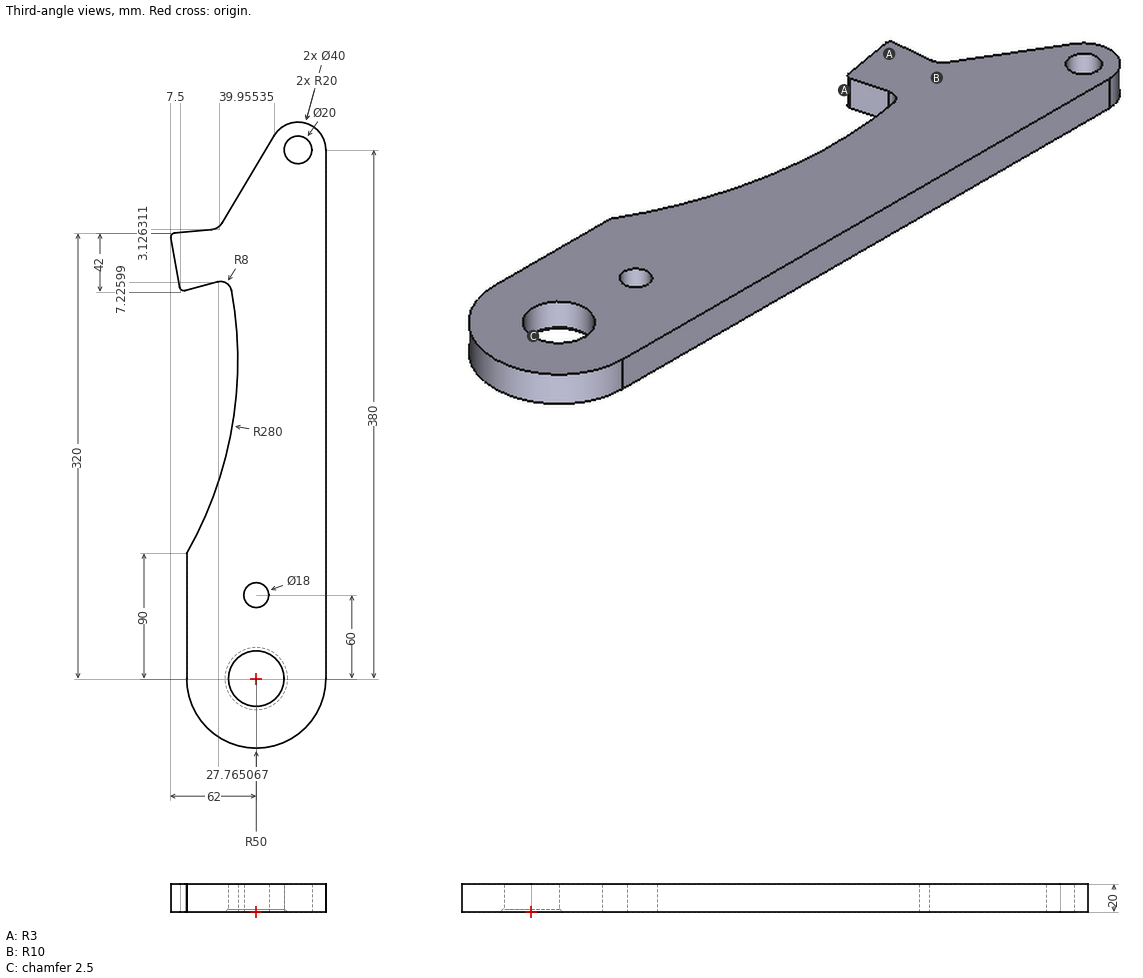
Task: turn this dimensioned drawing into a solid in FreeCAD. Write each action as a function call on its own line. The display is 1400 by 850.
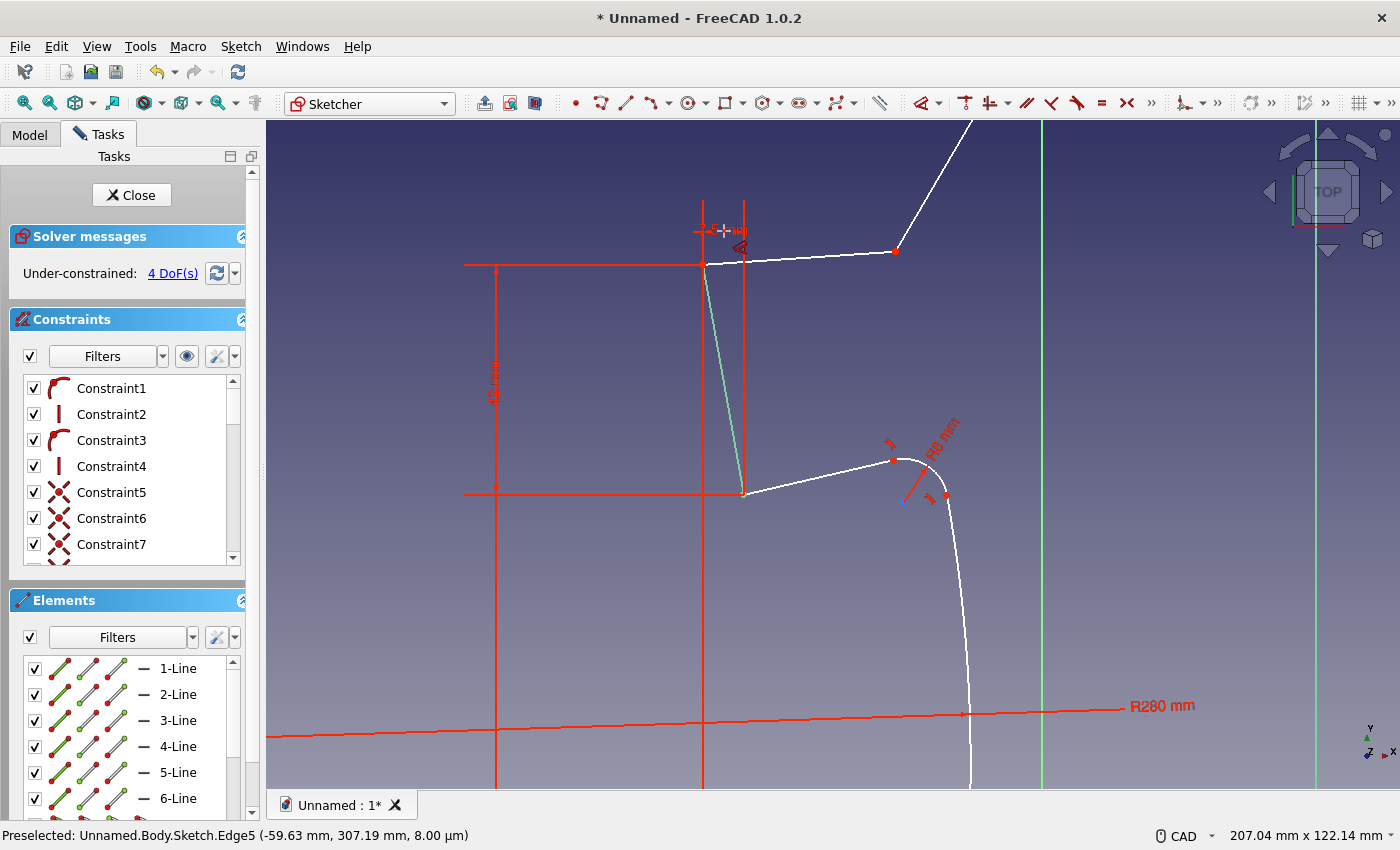
click(789, 484)
click(710, 477)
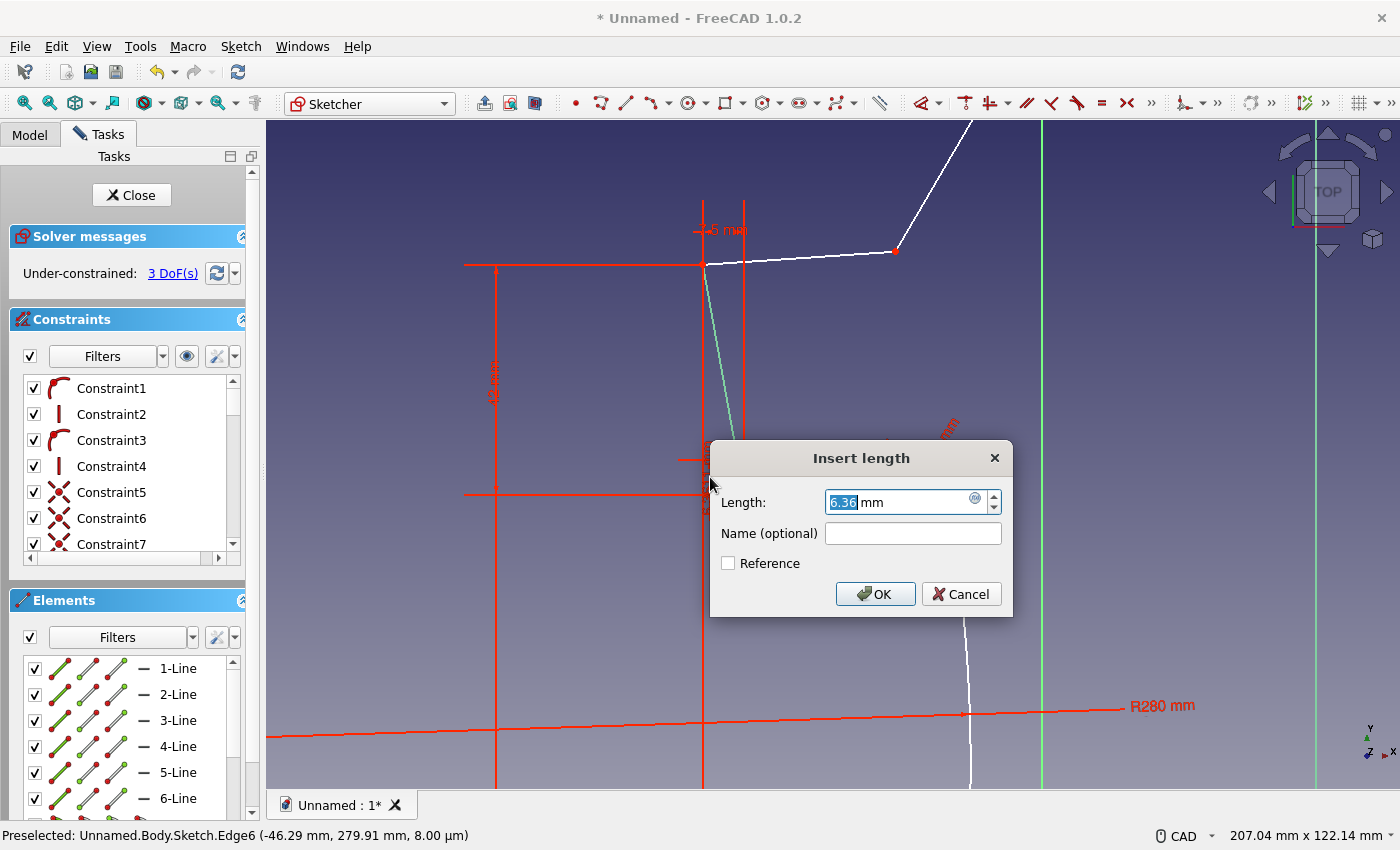
text(7.22599)
key(Return)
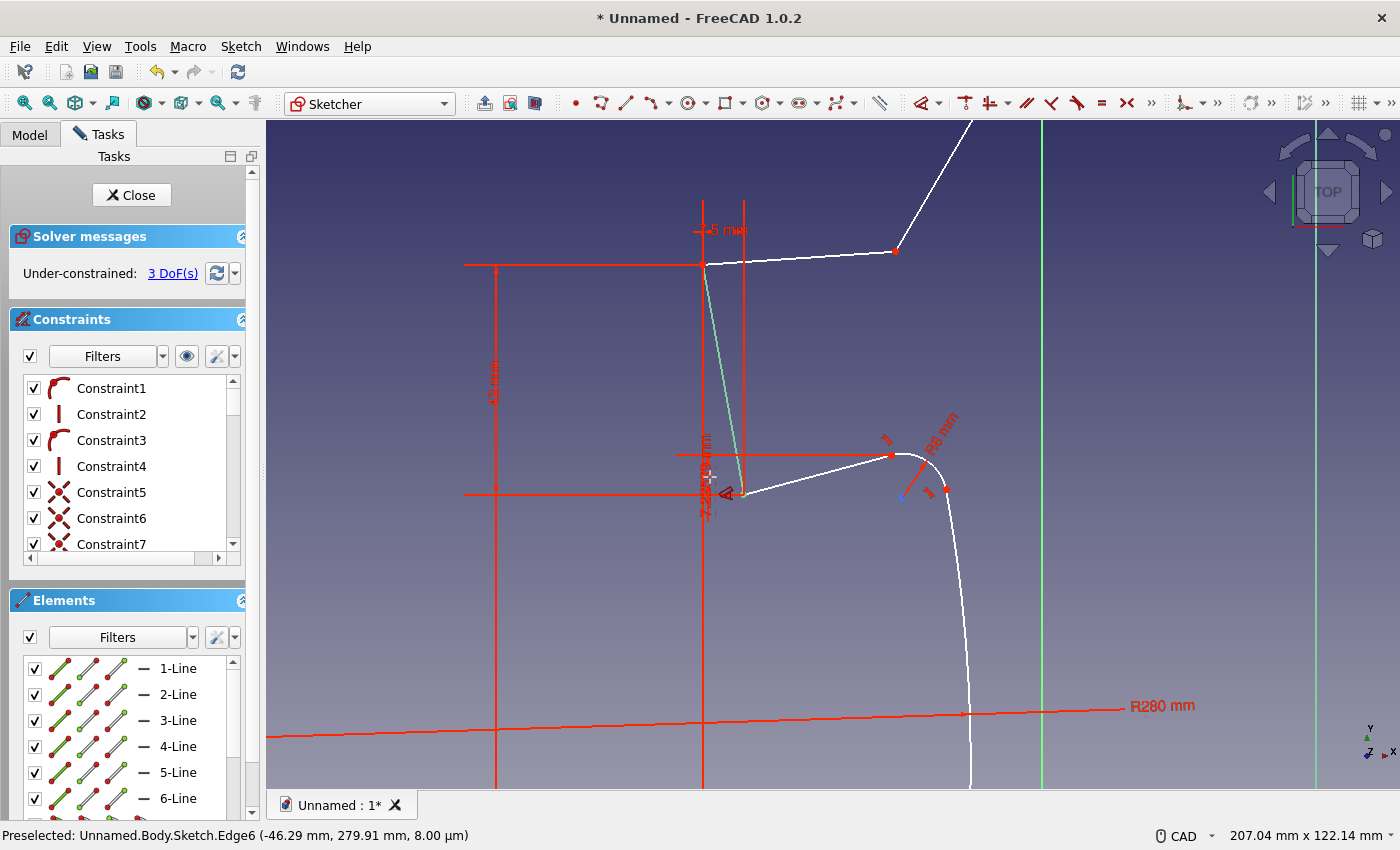
scroll(716, 334, down, 9)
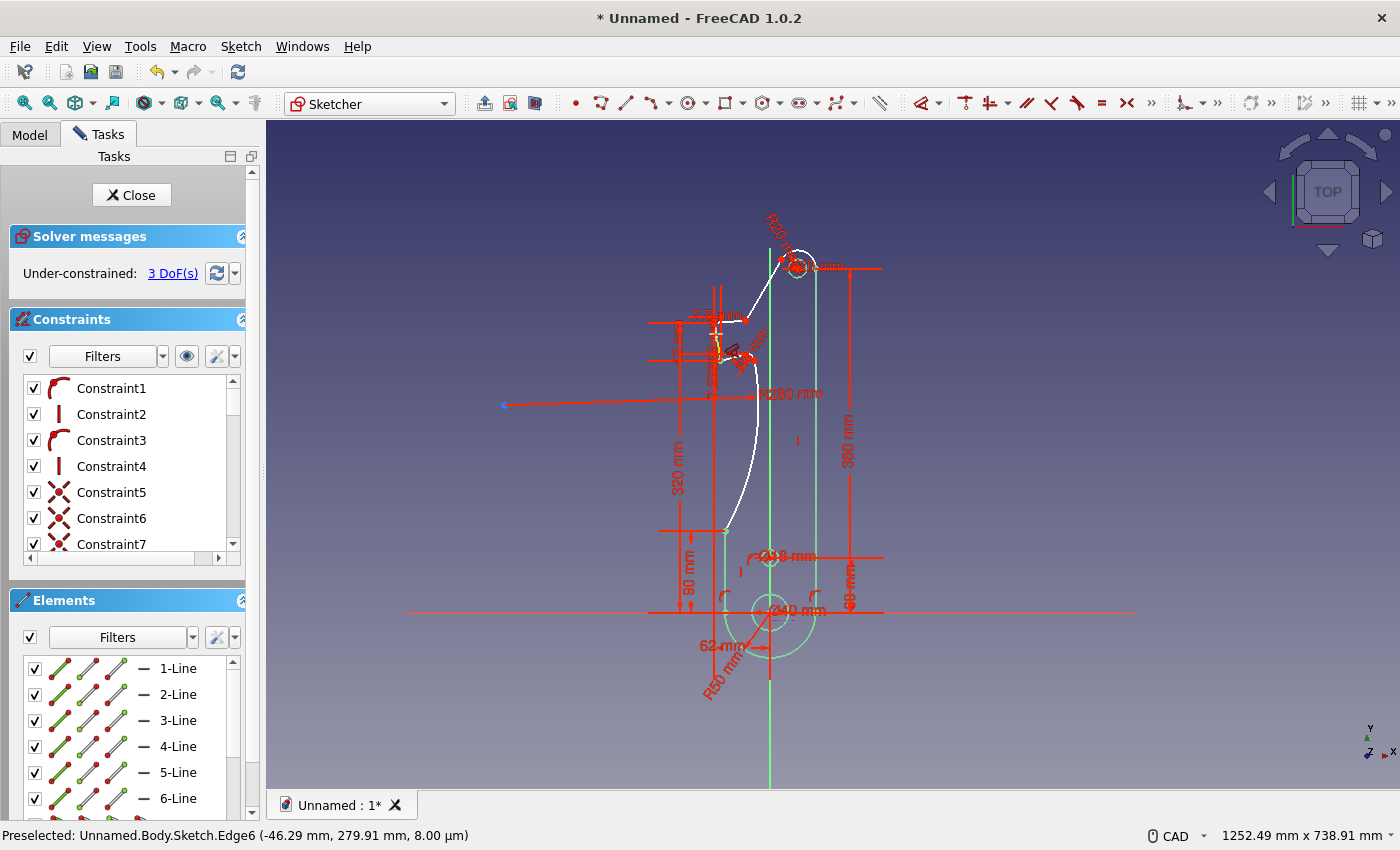
click(753, 308)
click(756, 201)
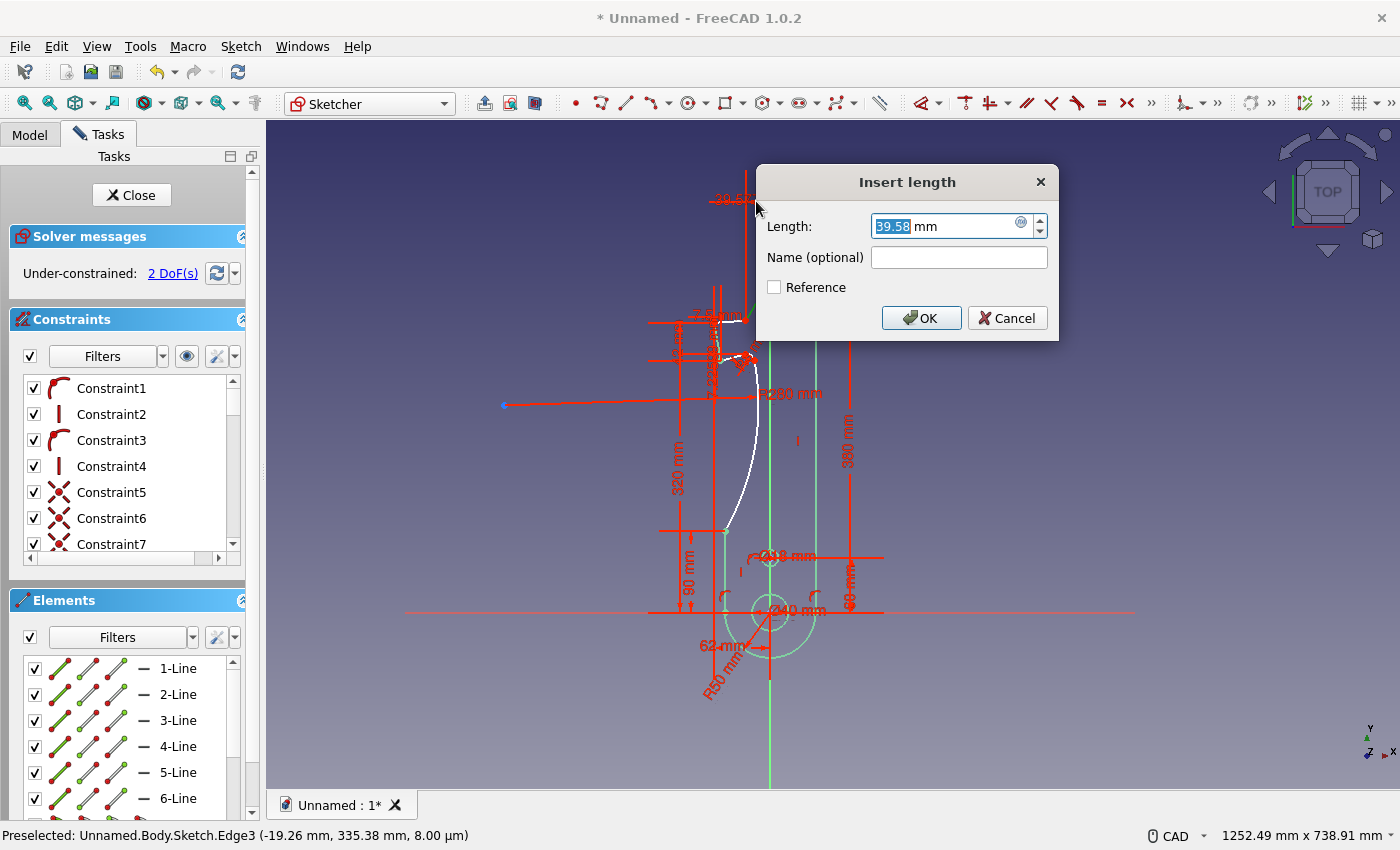
text(39.95535)
key(Return)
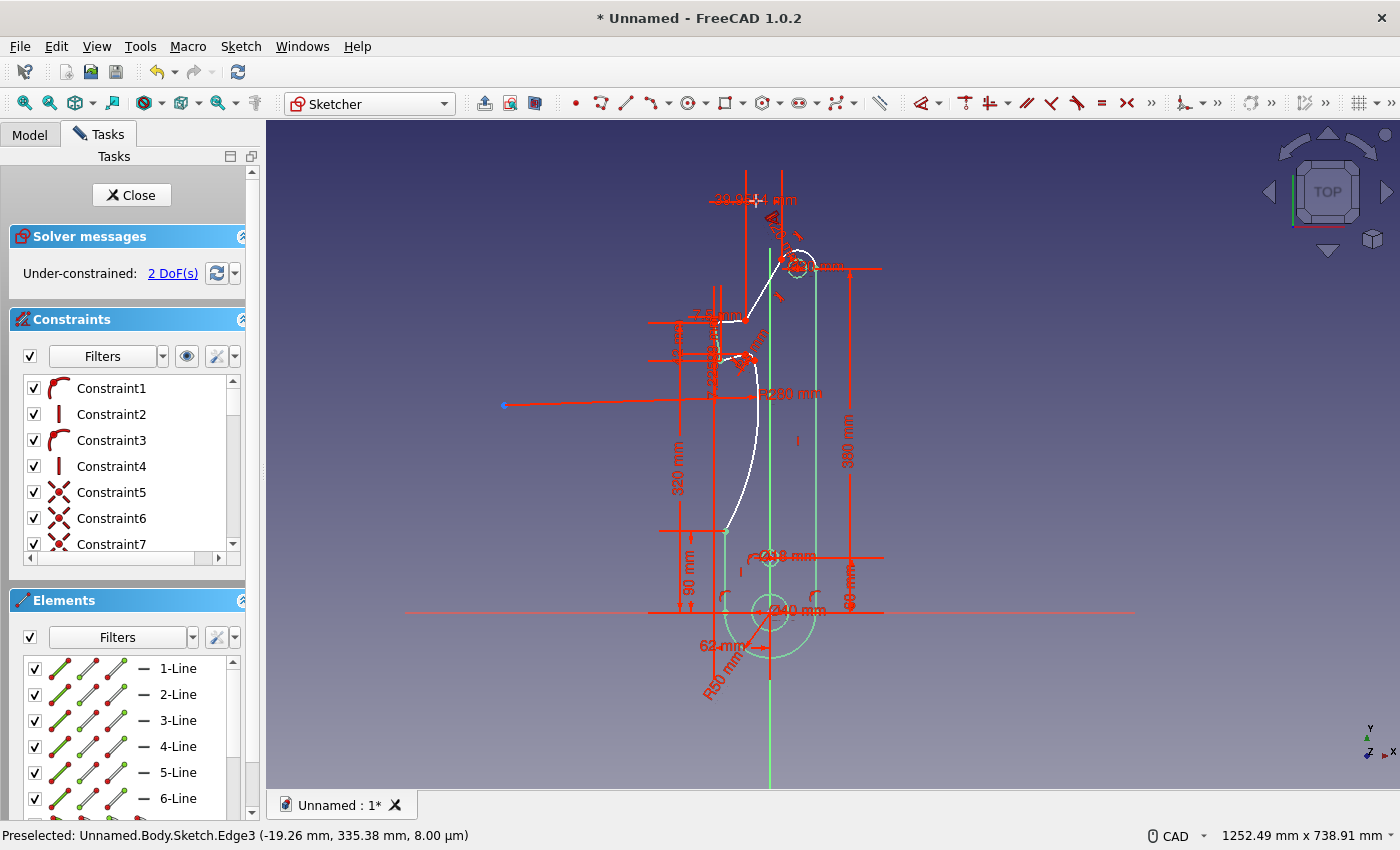
scroll(736, 321, up, 14)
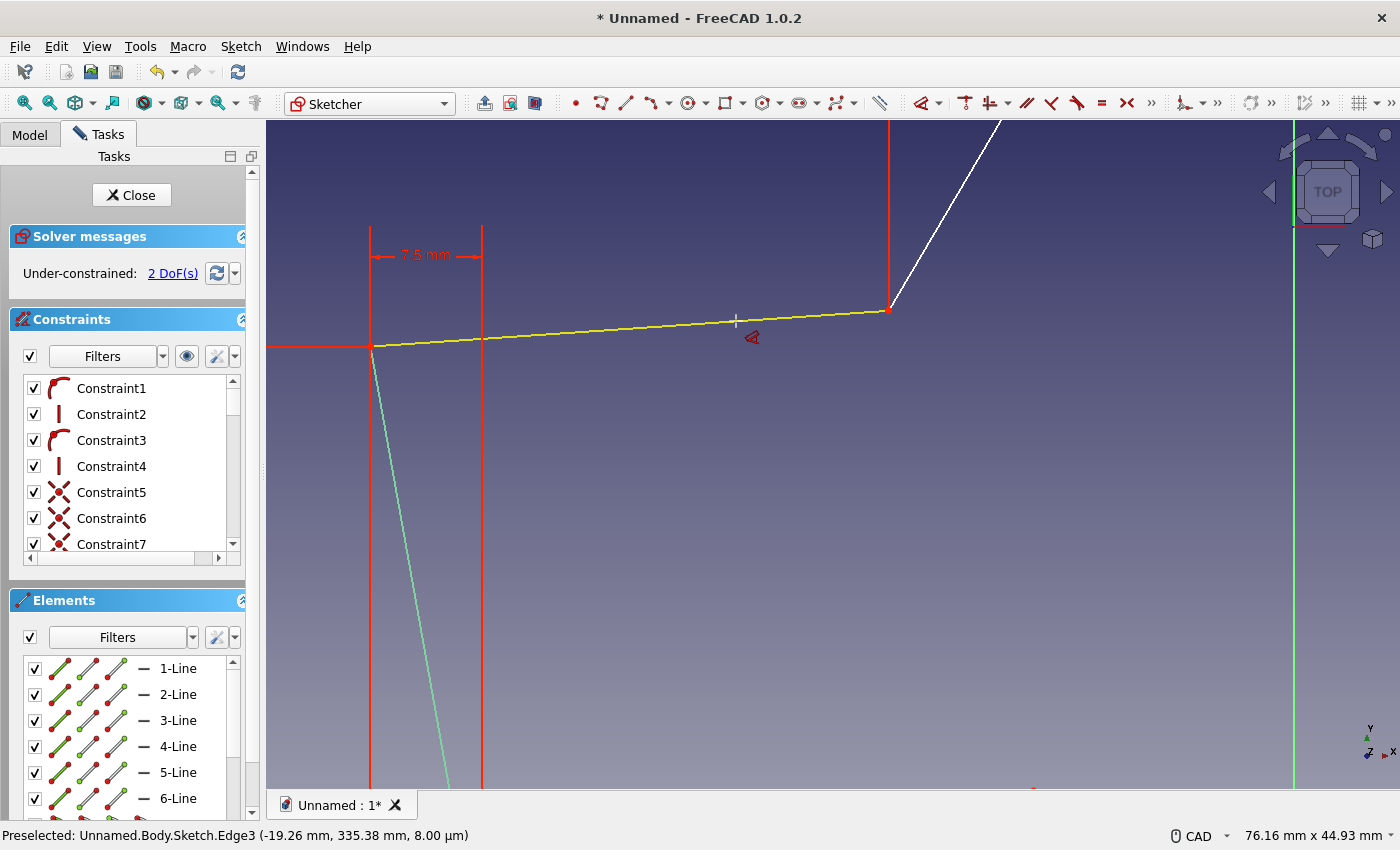
click(733, 322)
click(336, 329)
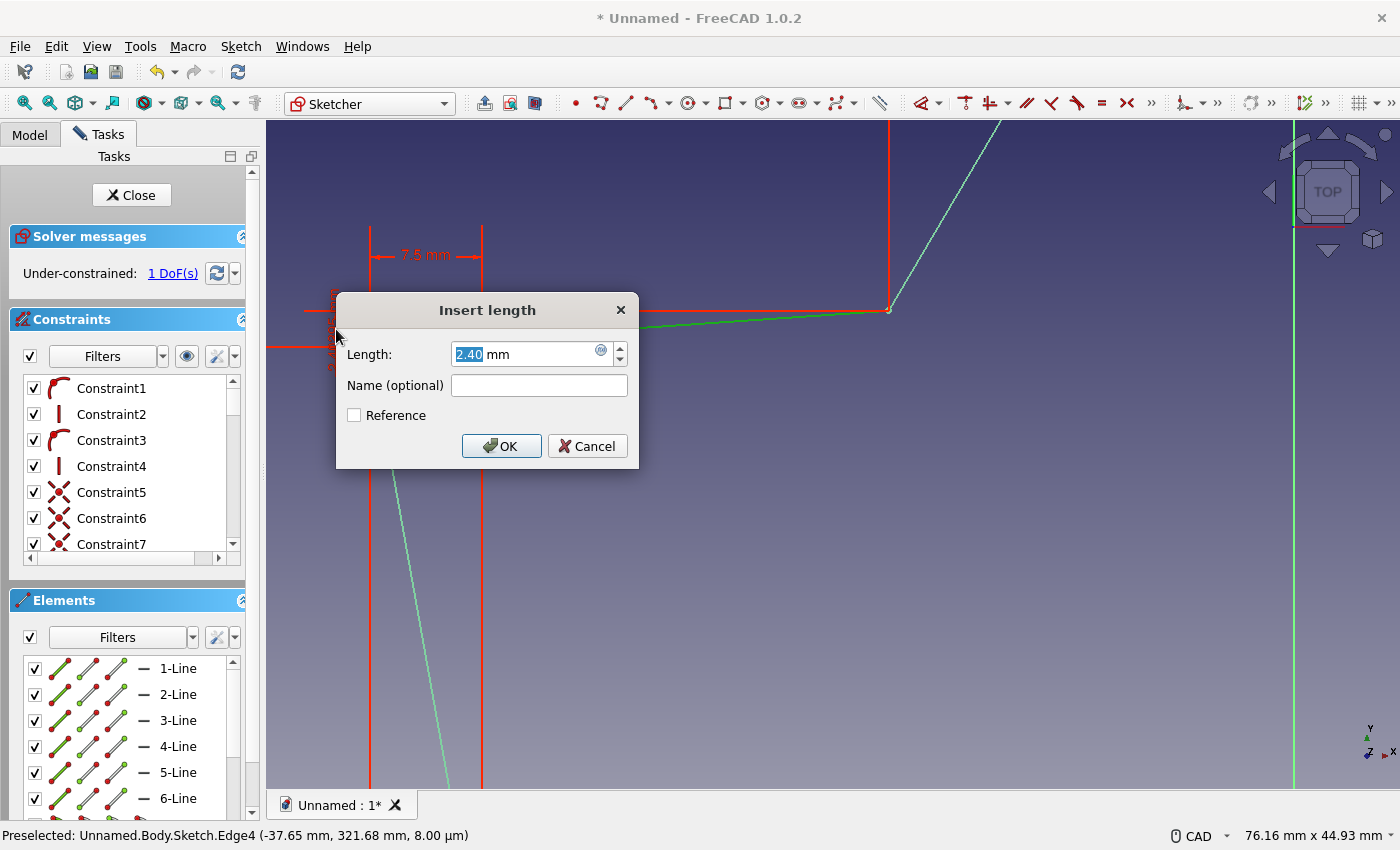
text(3.126311)
key(Return)